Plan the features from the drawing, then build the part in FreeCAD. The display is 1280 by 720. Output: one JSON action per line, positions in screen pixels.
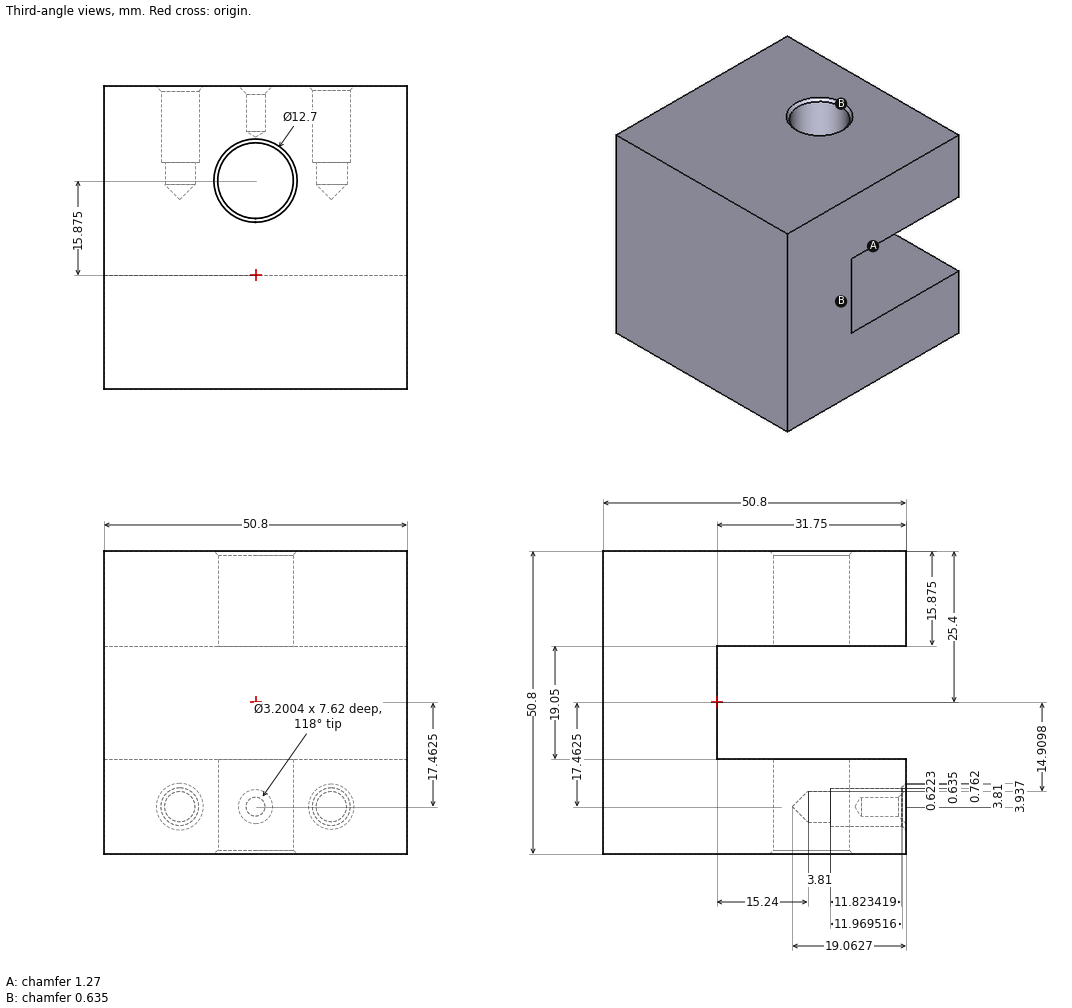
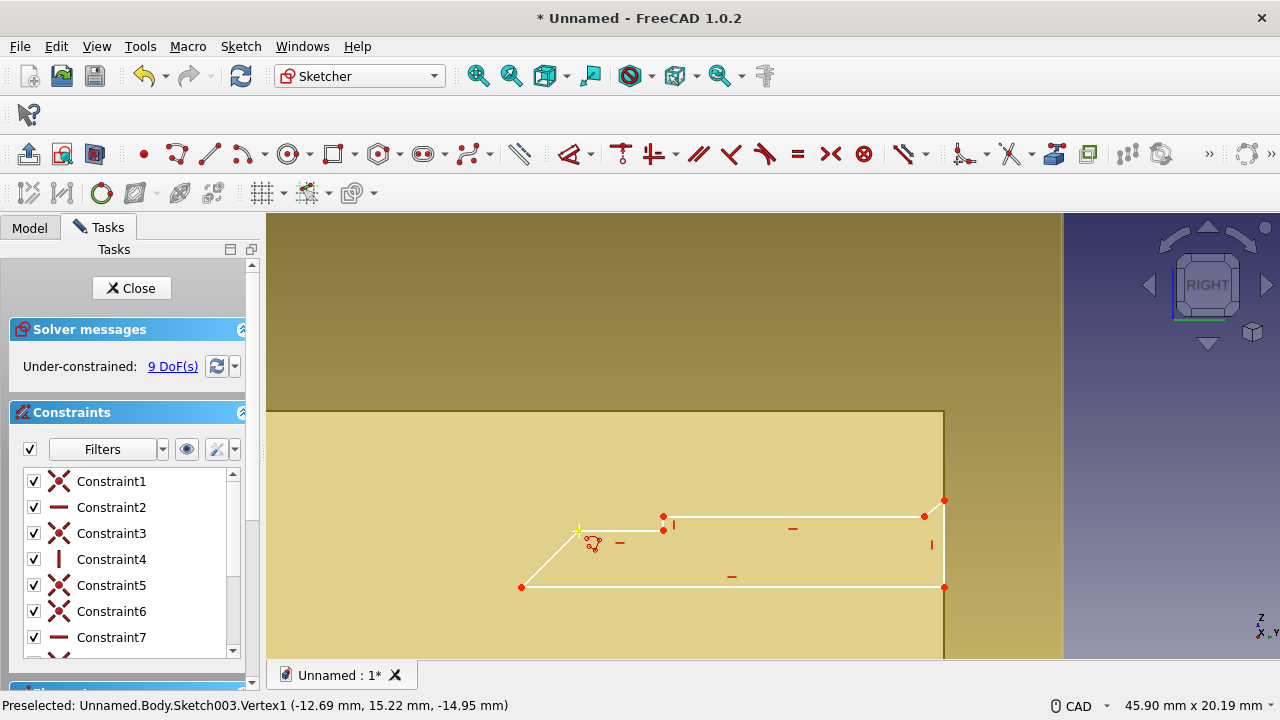
{"action": "left_click", "coordinate": [210, 154]}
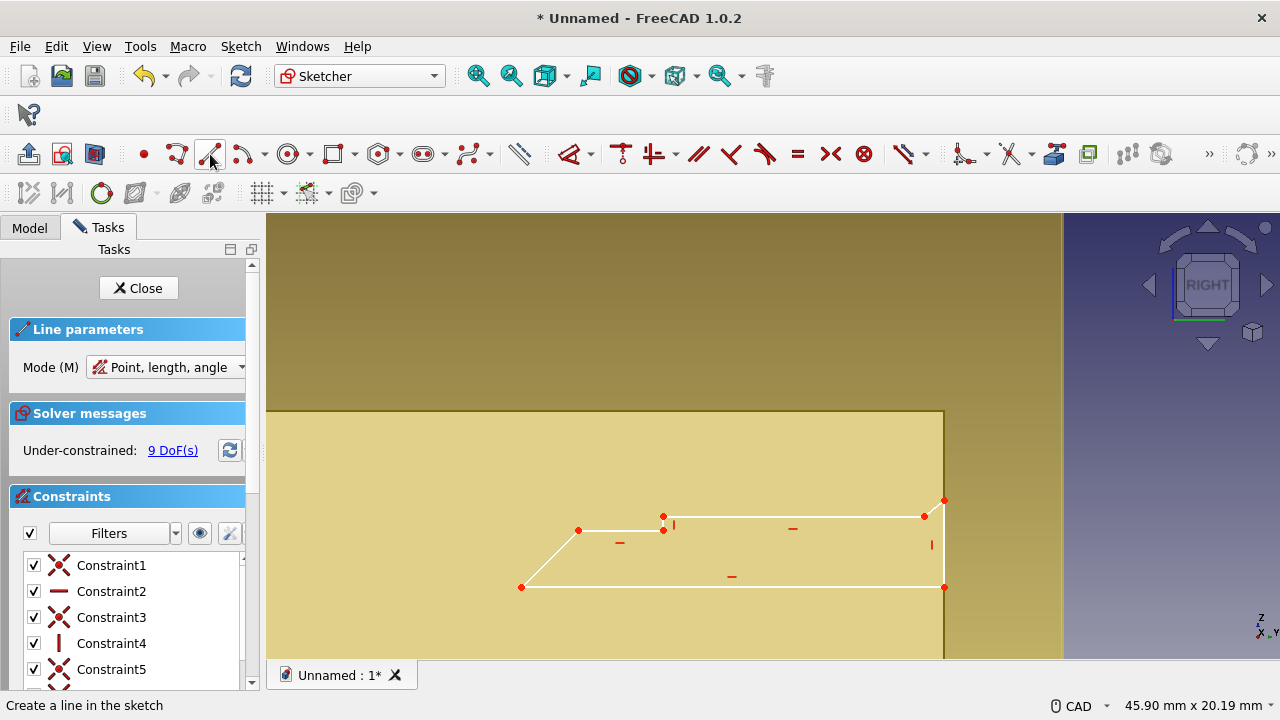
{"action": "left_click", "coordinate": [480, 586]}
{"action": "left_click", "coordinate": [354, 586]}
{"action": "key", "text": "Escape"}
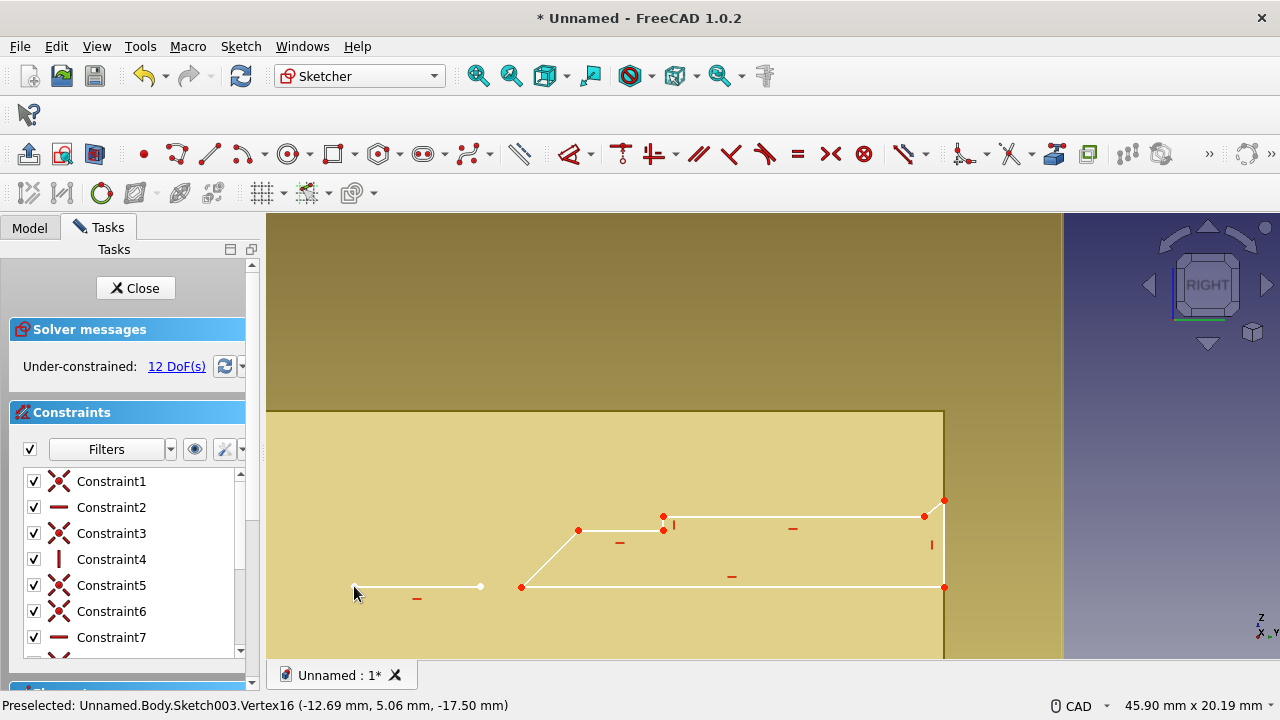
{"action": "left_click", "coordinate": [442, 587]}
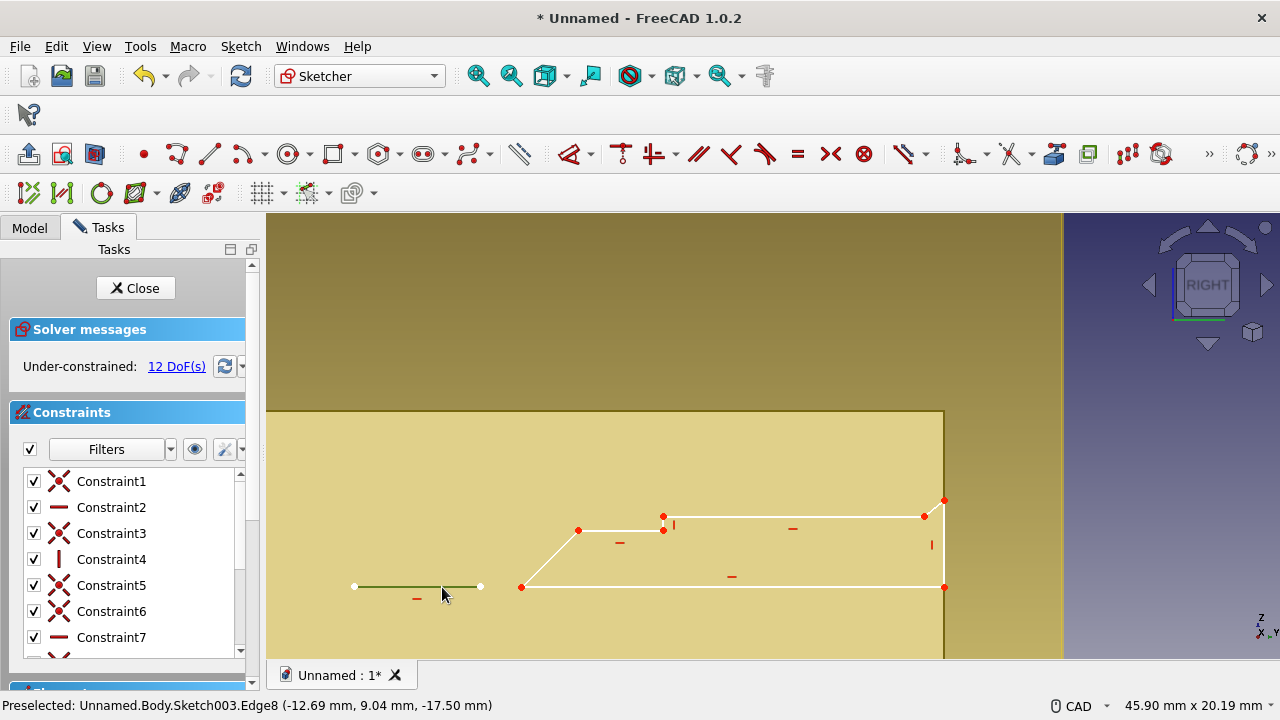
{"action": "left_click", "coordinate": [520, 154]}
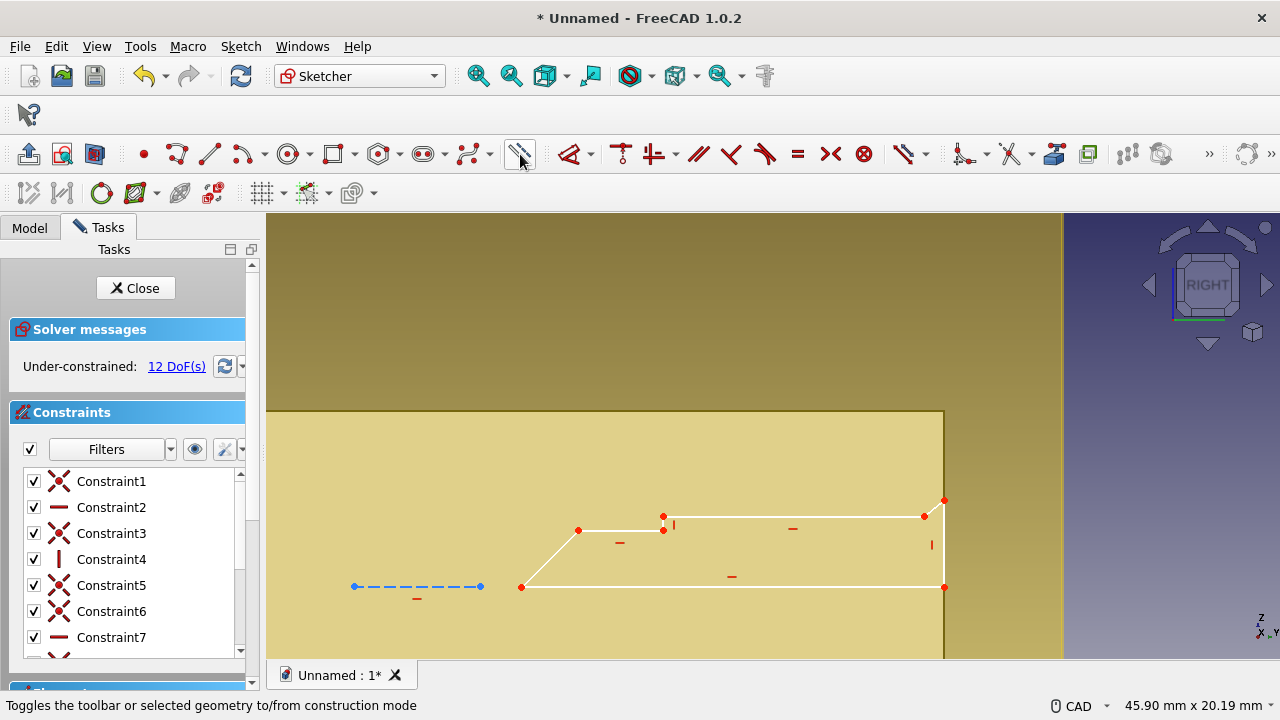
{"action": "left_click", "coordinate": [568, 154]}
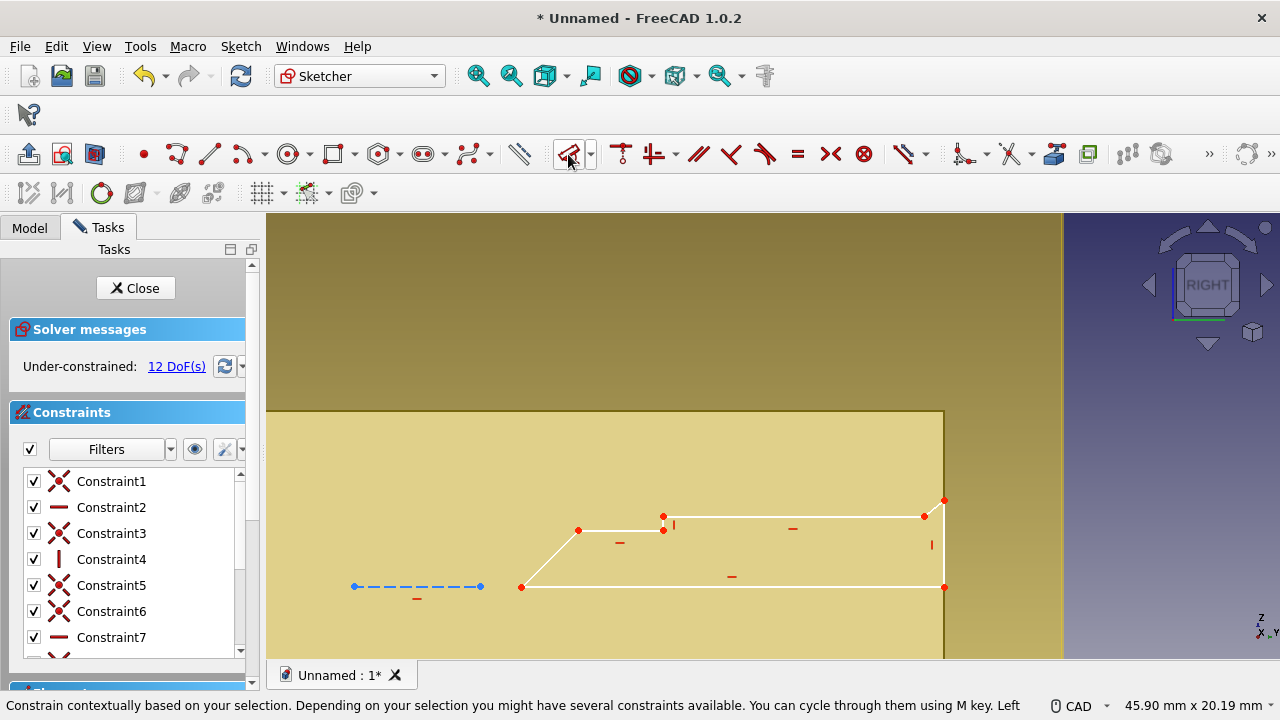
{"action": "left_click", "coordinate": [638, 531]}
{"action": "left_click", "coordinate": [621, 565]}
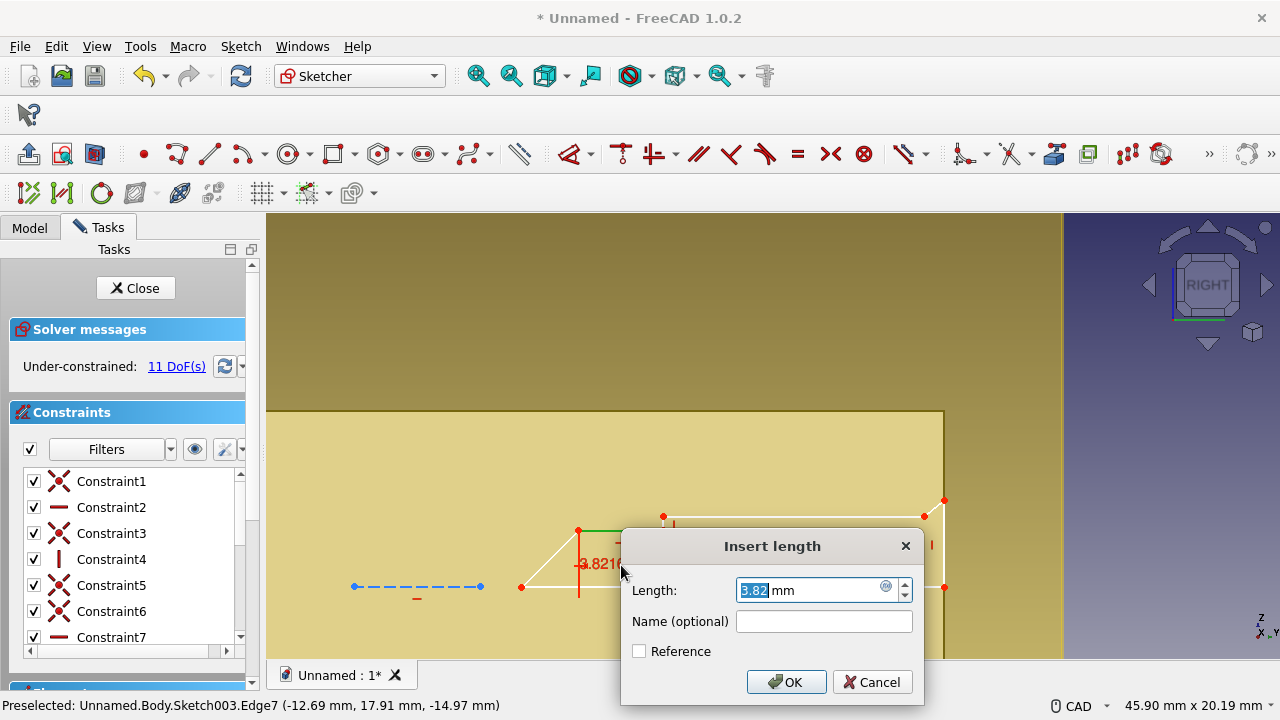
{"action": "type", "text": "3.81"}
{"action": "key", "text": "Return"}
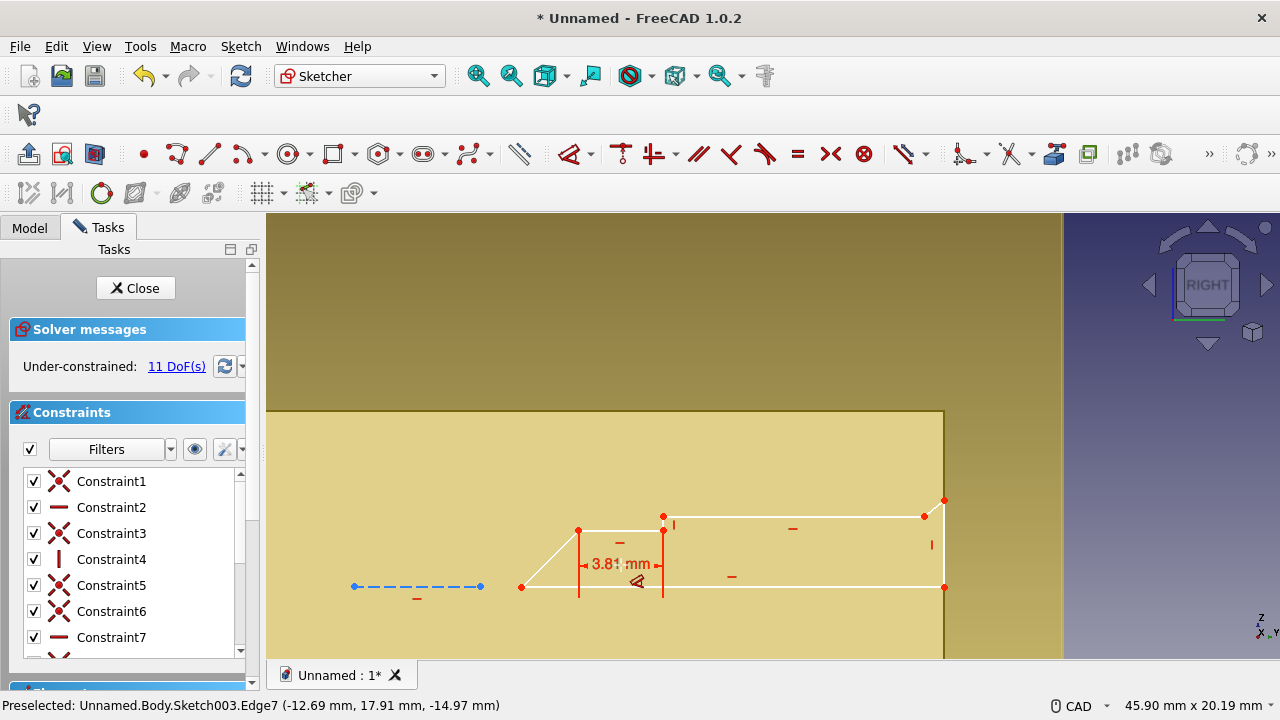
{"action": "left_click", "coordinate": [944, 561]}
{"action": "left_click", "coordinate": [978, 544]}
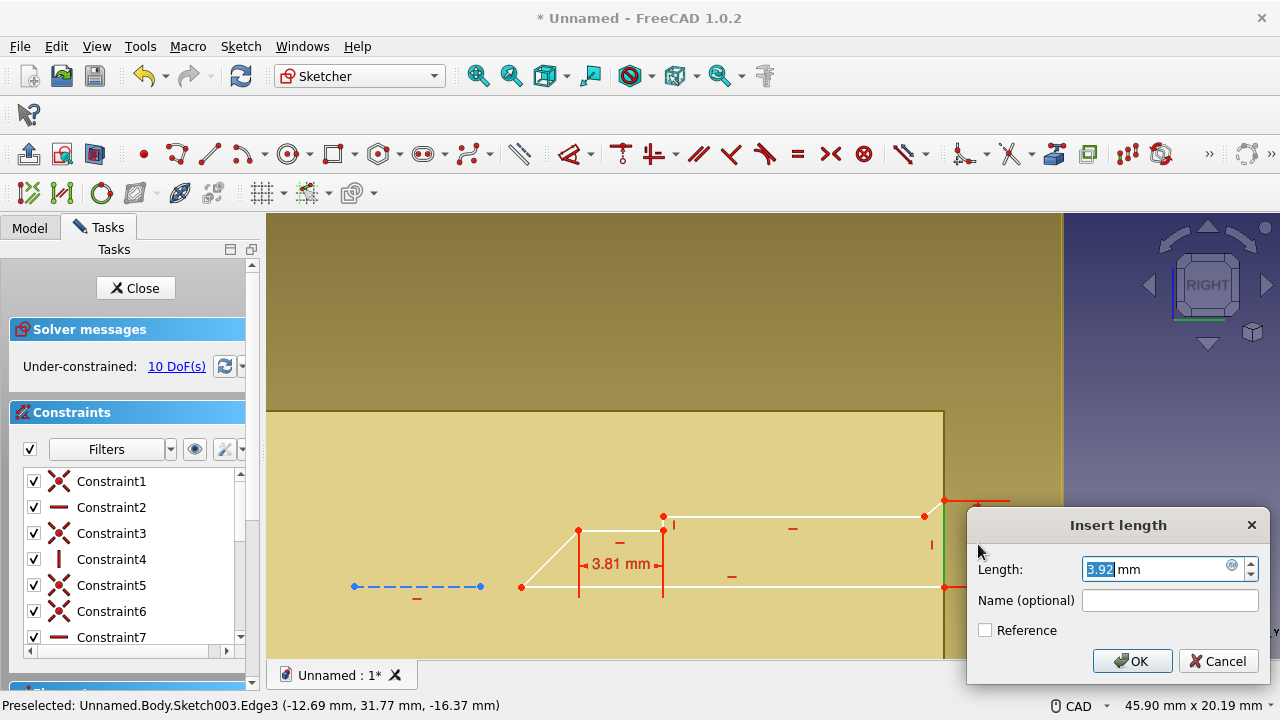
{"action": "type", "text": "3.937"}
{"action": "key", "text": "Return"}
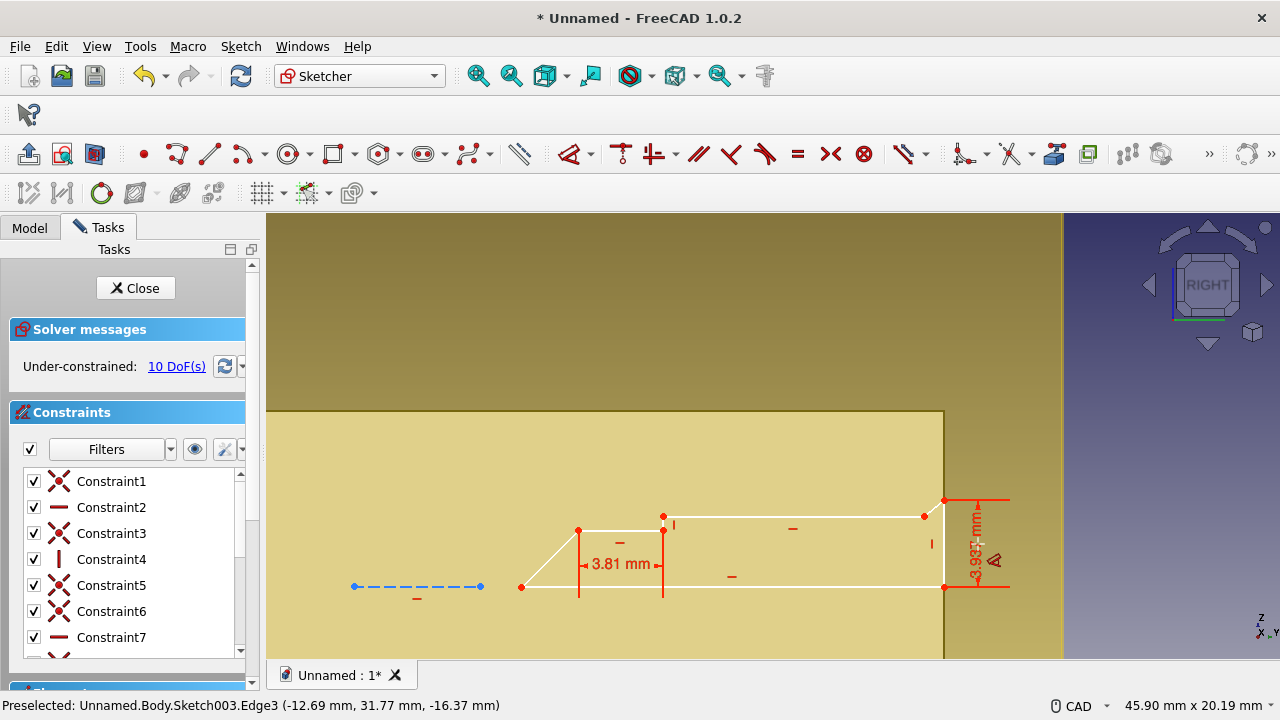
{"action": "scroll", "coordinate": [663, 524], "scroll_direction": "up", "scroll_amount": 6}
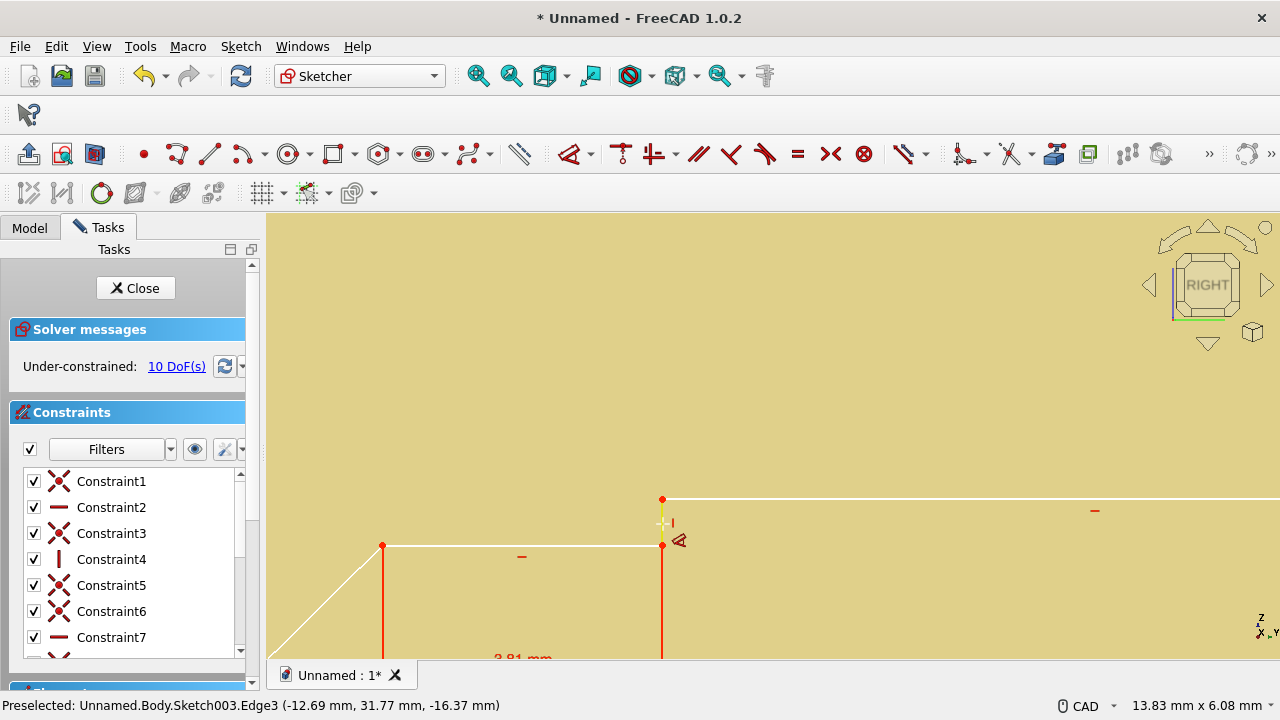
{"action": "left_click", "coordinate": [662, 522]}
{"action": "left_click", "coordinate": [696, 522]}